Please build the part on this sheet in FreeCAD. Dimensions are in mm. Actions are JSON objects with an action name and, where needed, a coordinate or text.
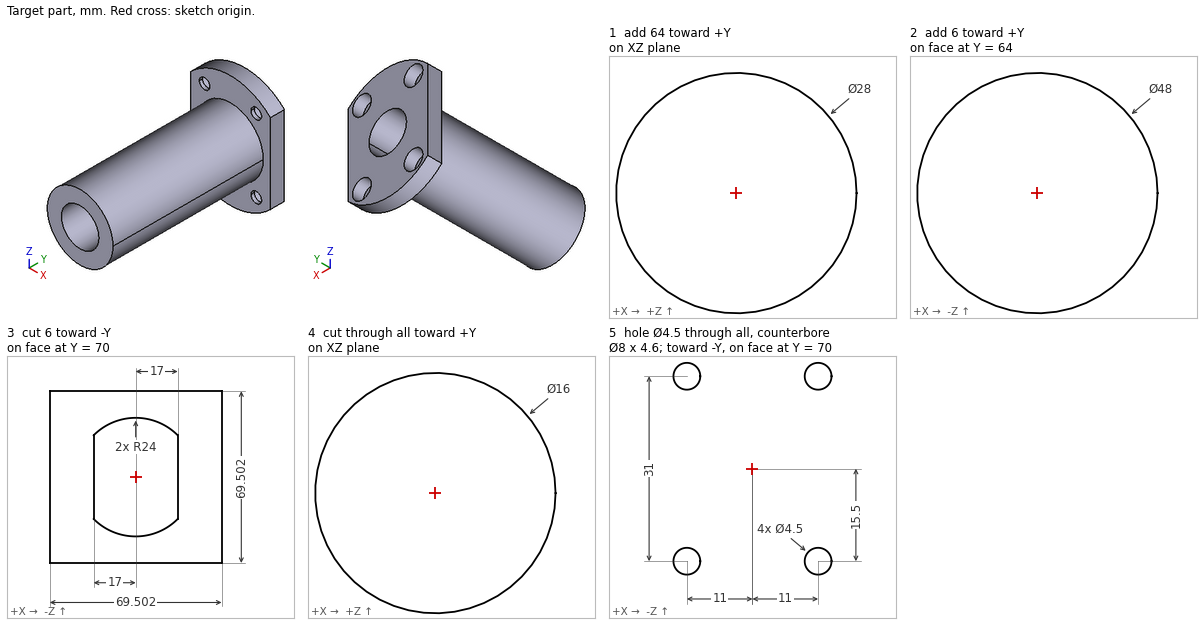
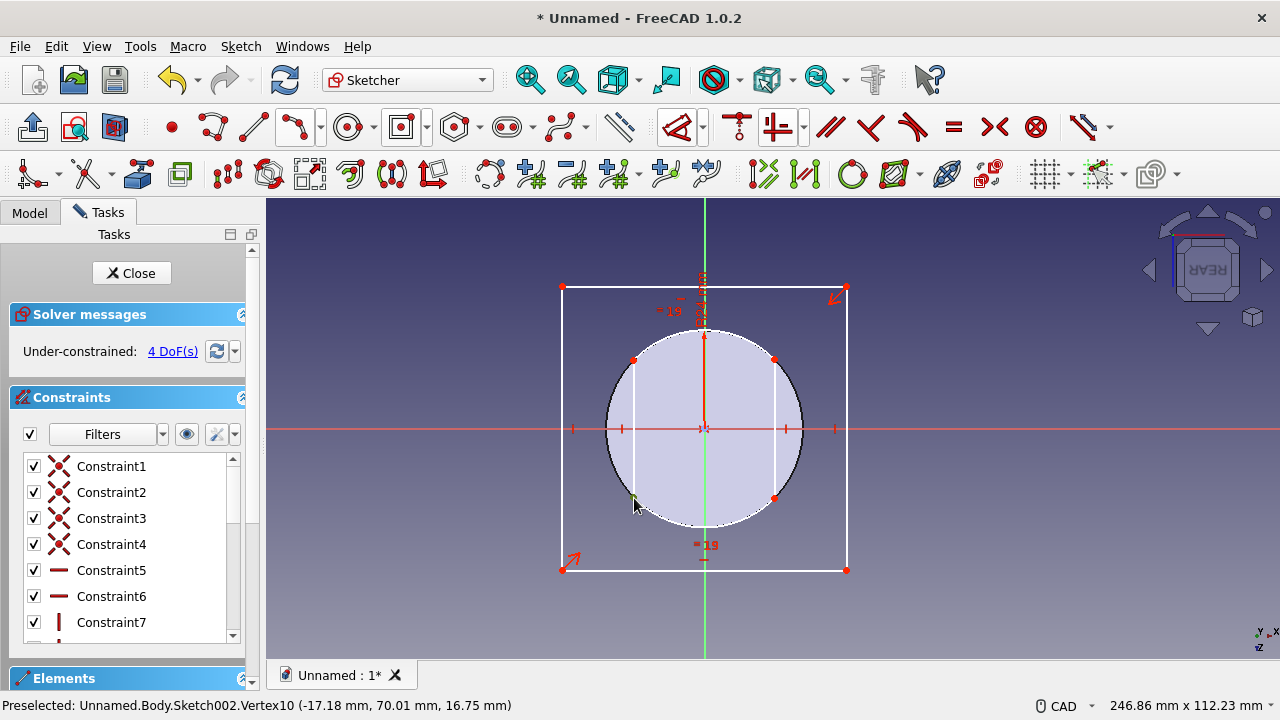
{"action": "key", "text": "l"}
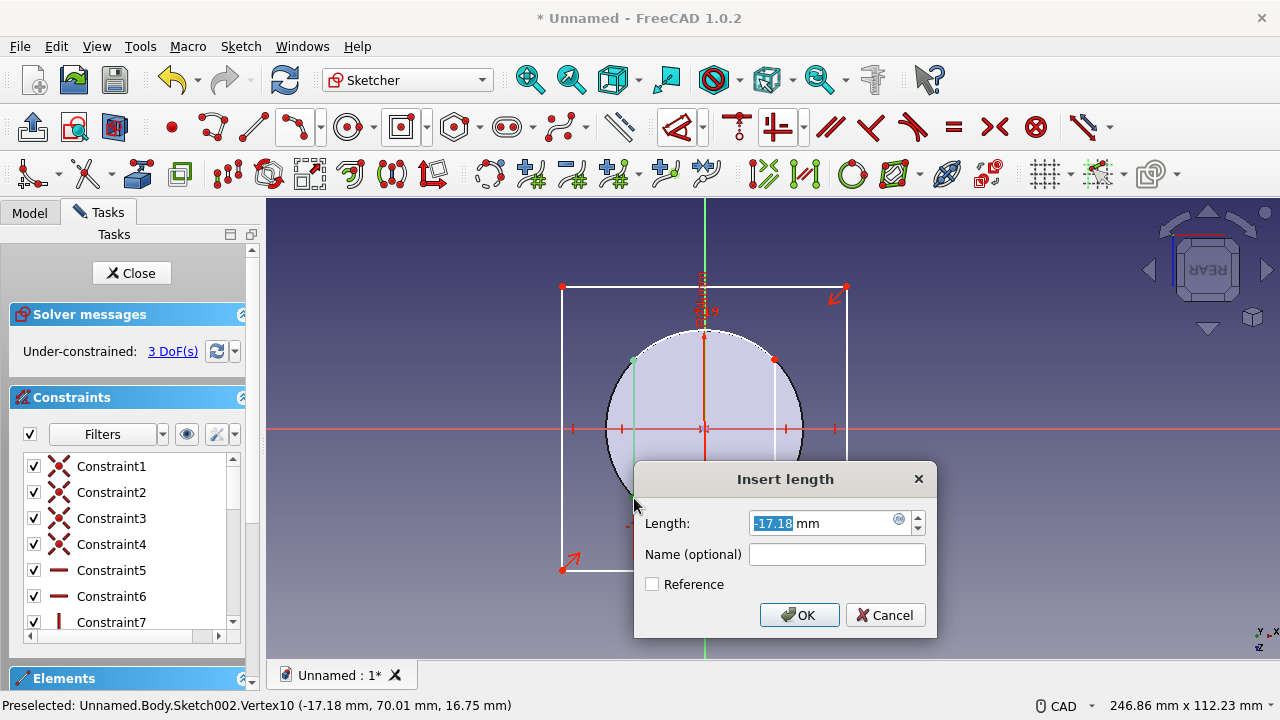
{"action": "type", "text": "-17"}
{"action": "key", "text": "Return"}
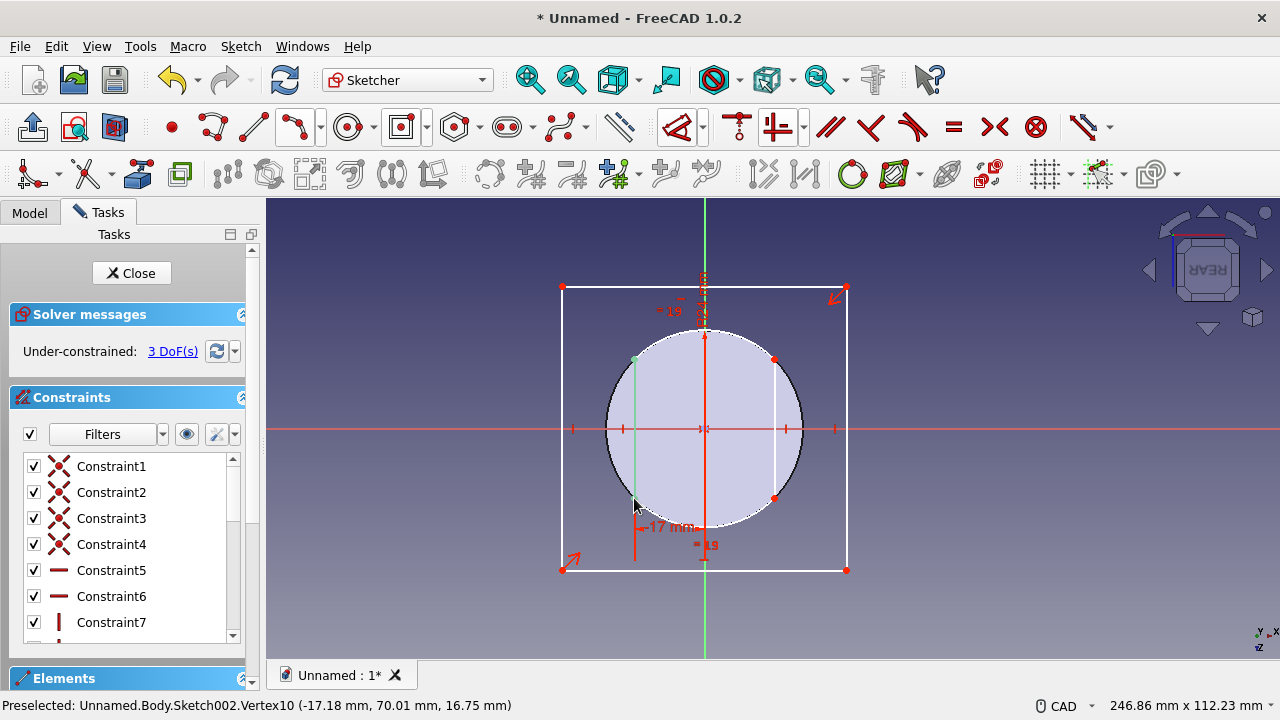
{"action": "left_click", "coordinate": [775, 360]}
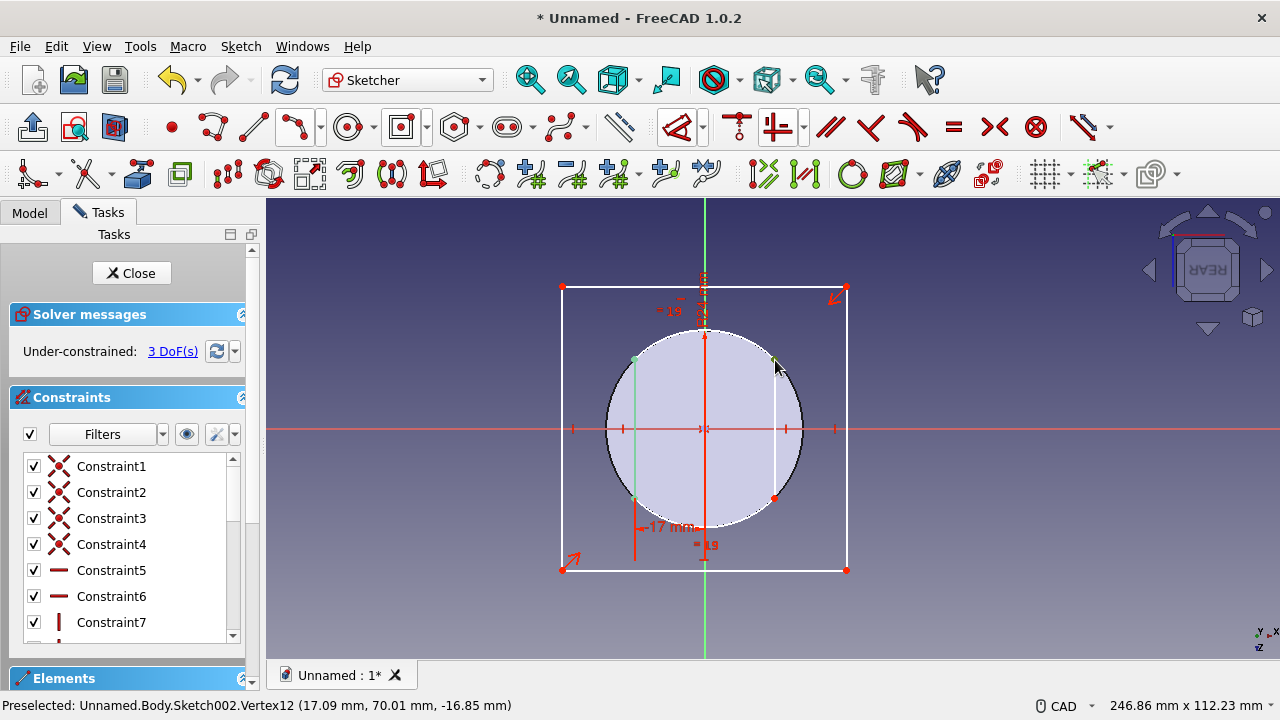
{"action": "key", "text": "l"}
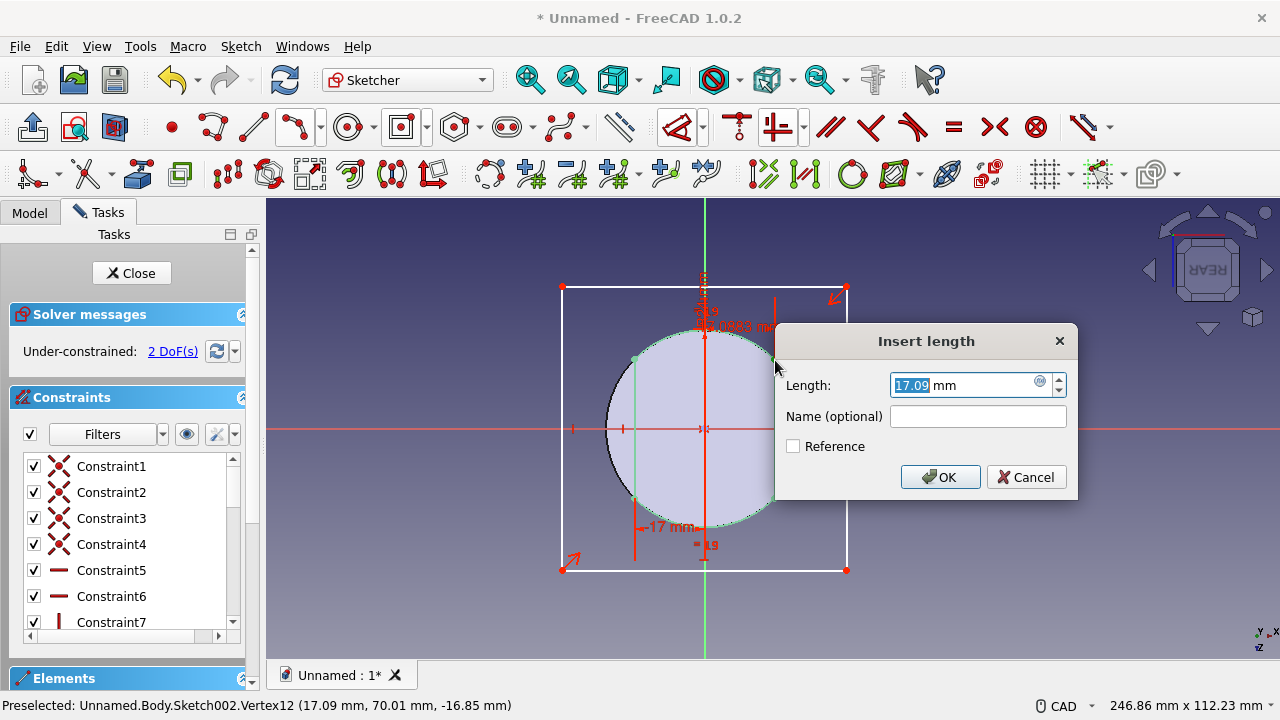
{"action": "type", "text": "17"}
{"action": "key", "text": "Return"}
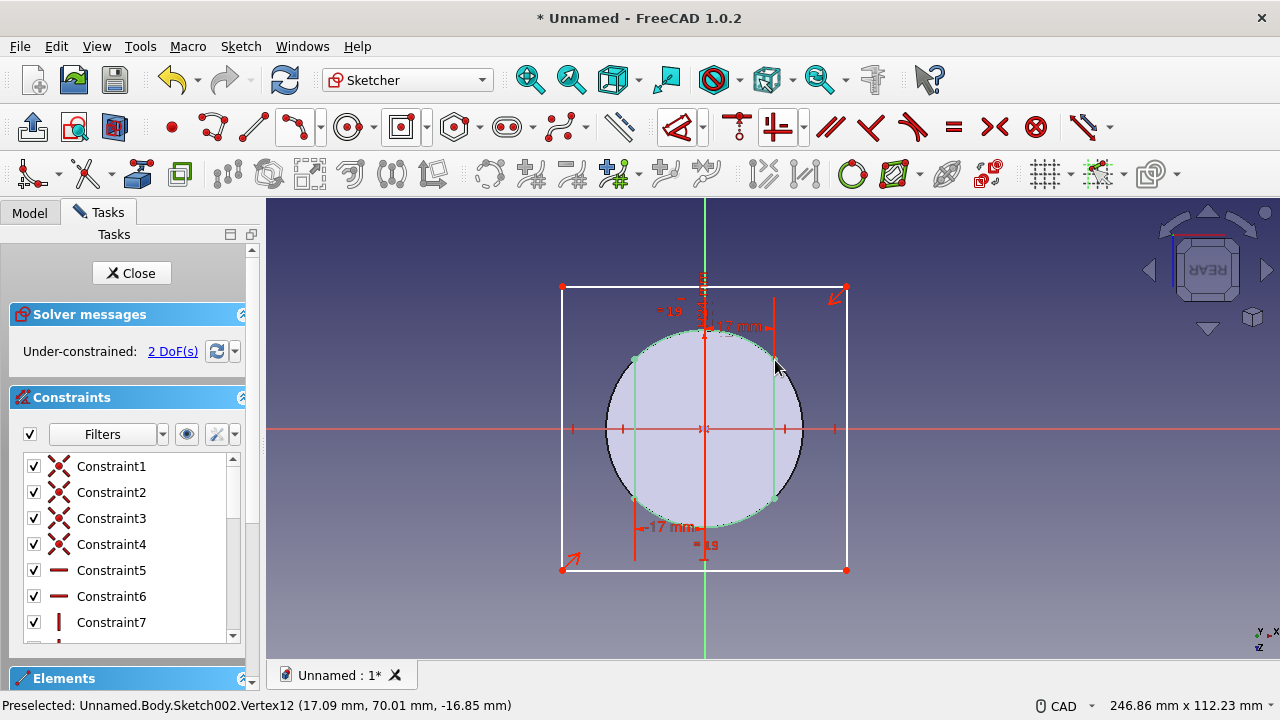
{"action": "left_click", "coordinate": [648, 571]}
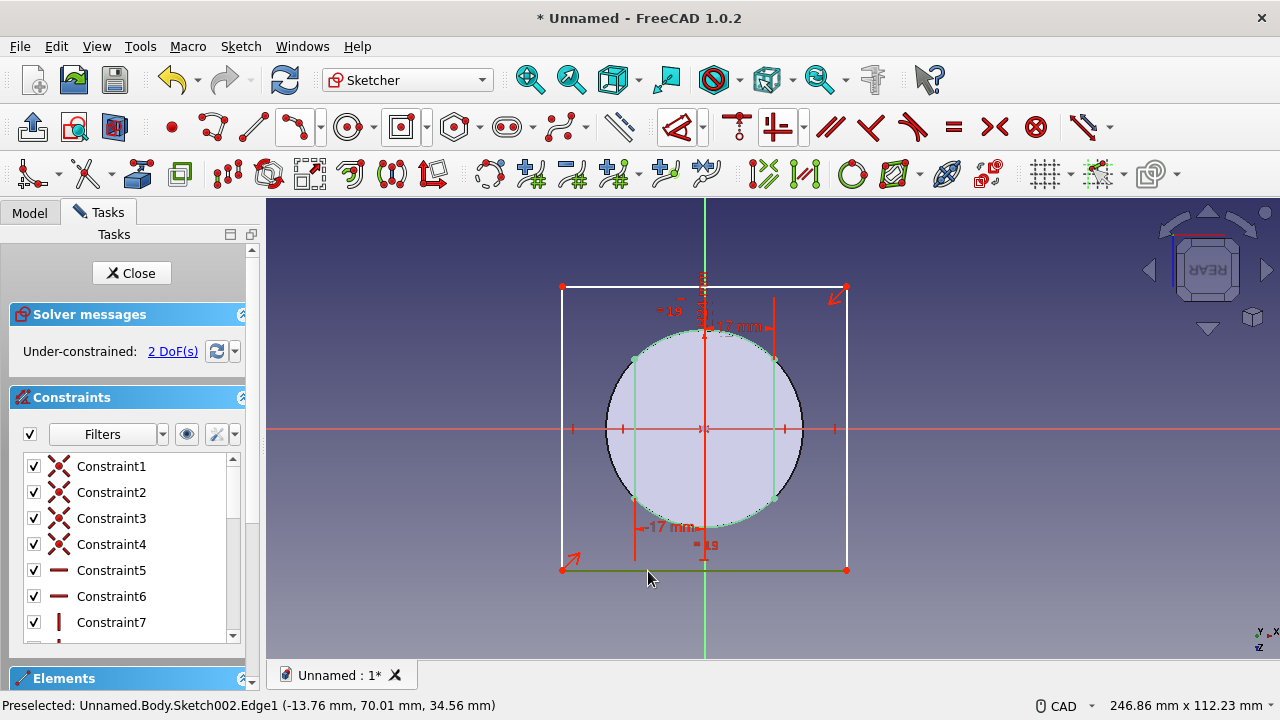
{"action": "left_click", "coordinate": [702, 128]}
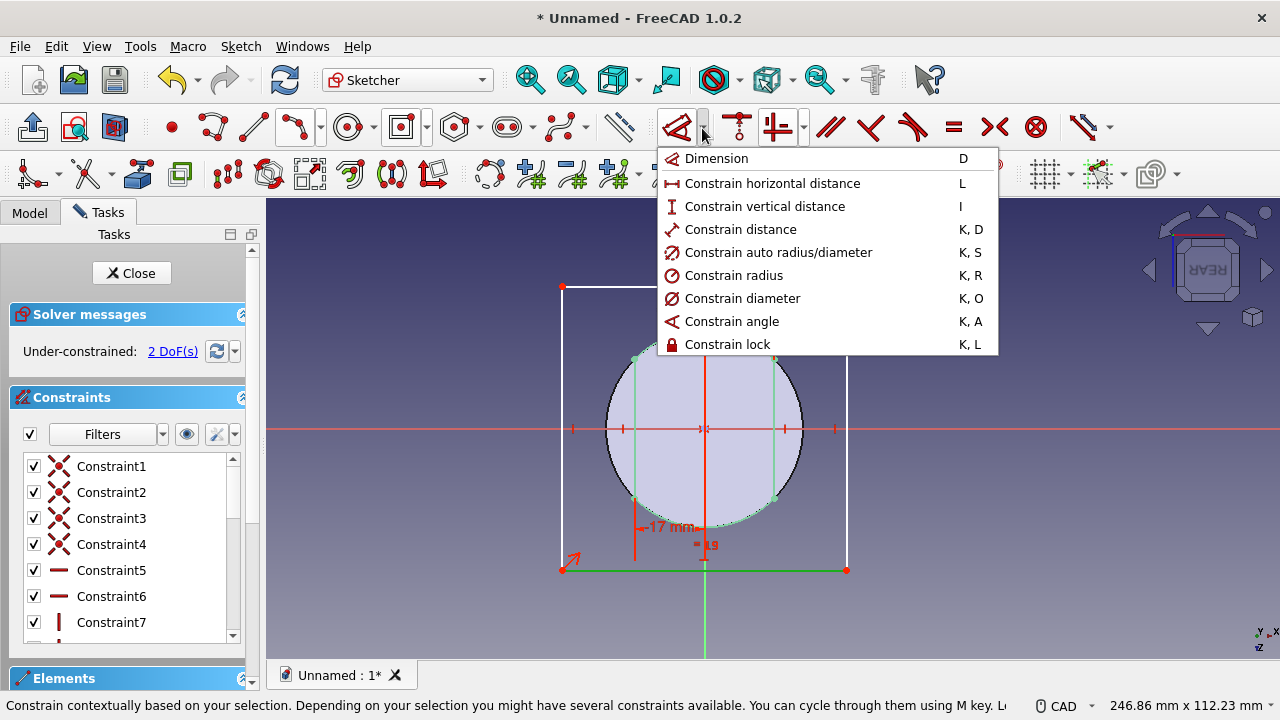
{"action": "left_click", "coordinate": [828, 184]}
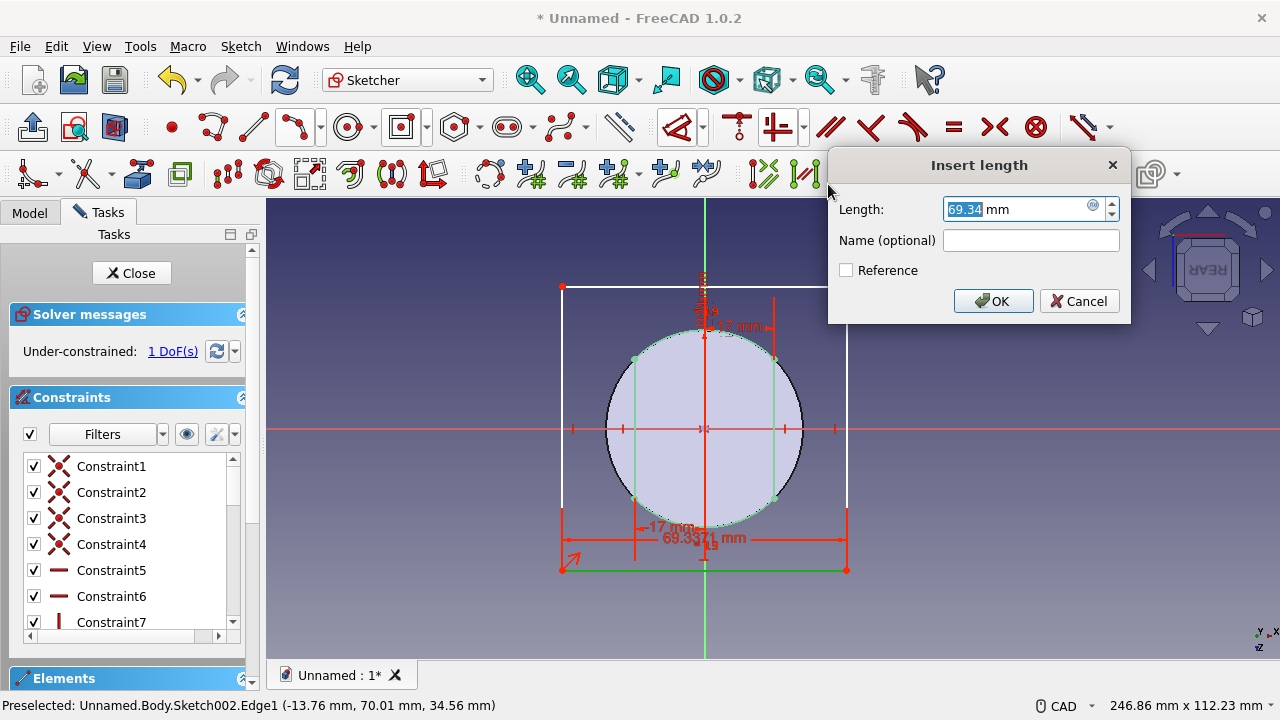
{"action": "type", "text": "69.502"}
{"action": "key", "text": "Return"}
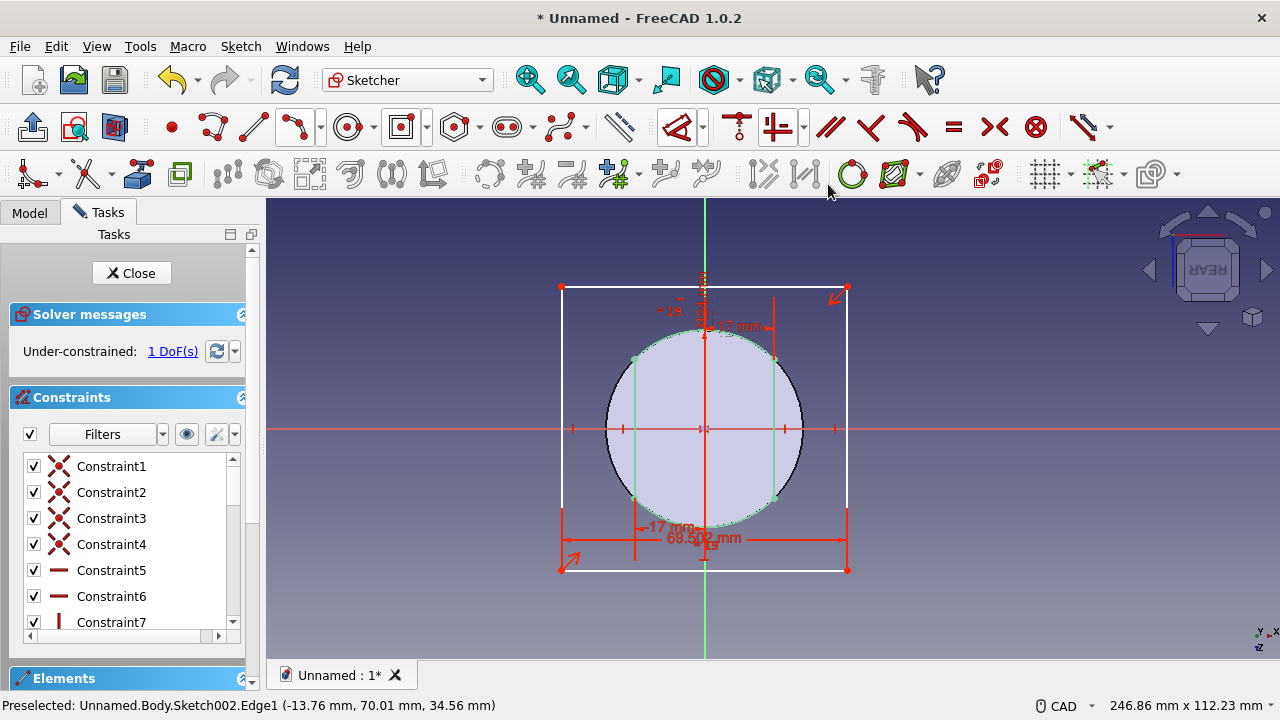
{"action": "left_click", "coordinate": [847, 486]}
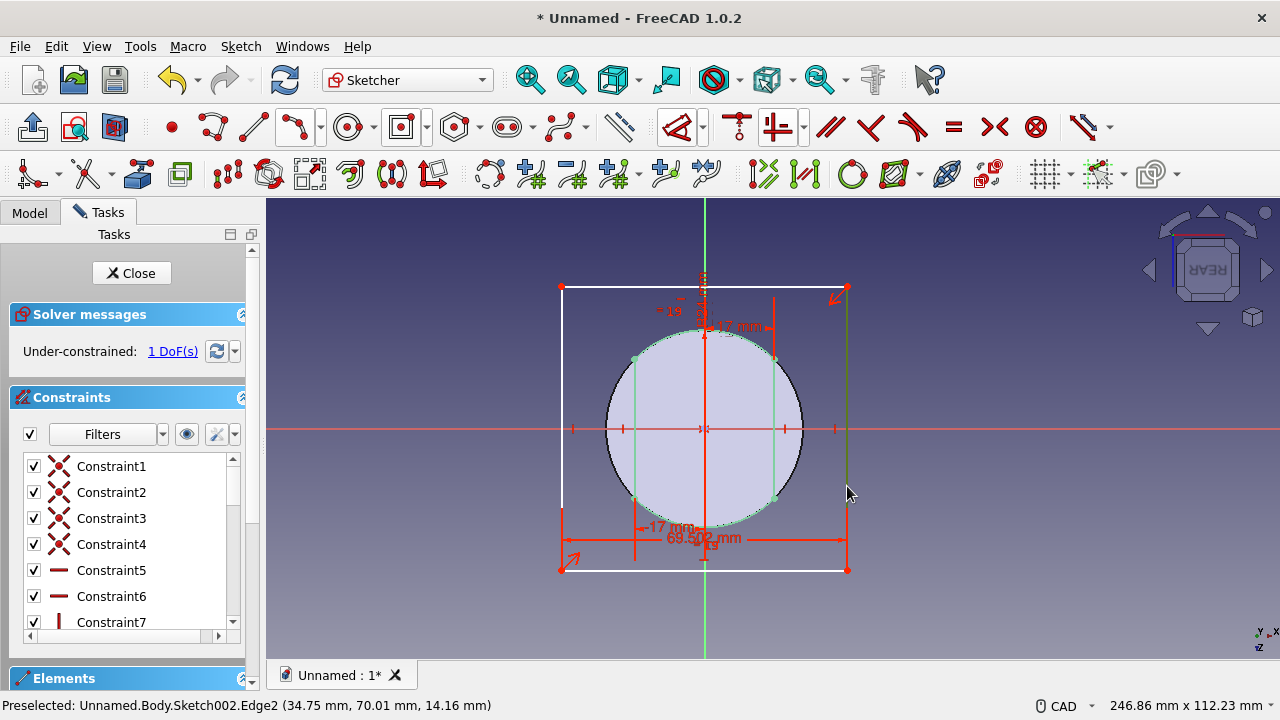
{"action": "key", "text": "i"}